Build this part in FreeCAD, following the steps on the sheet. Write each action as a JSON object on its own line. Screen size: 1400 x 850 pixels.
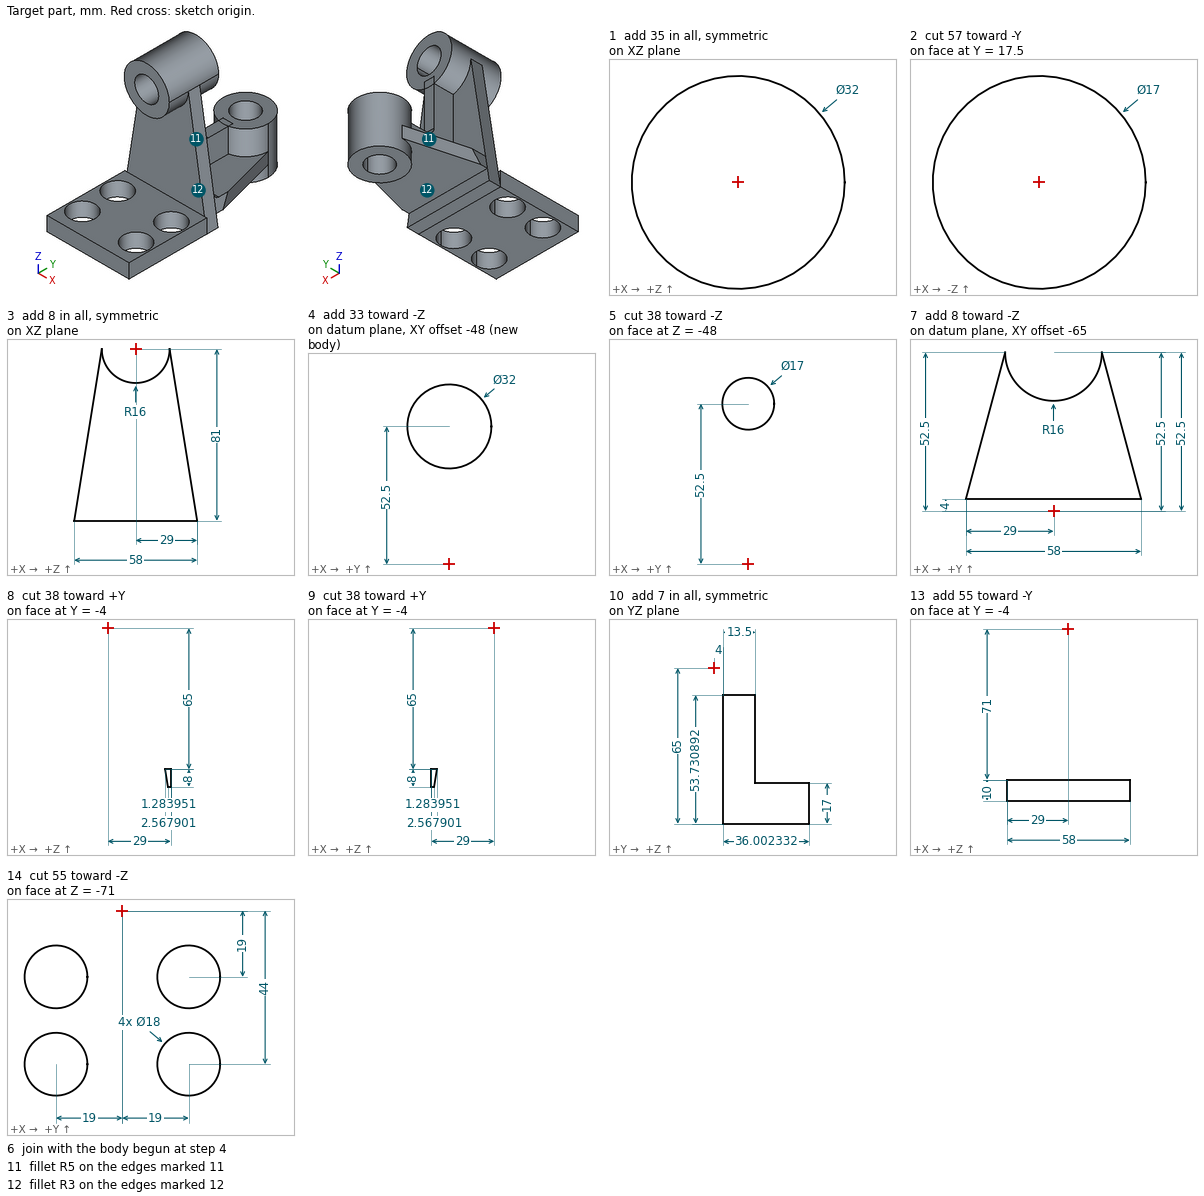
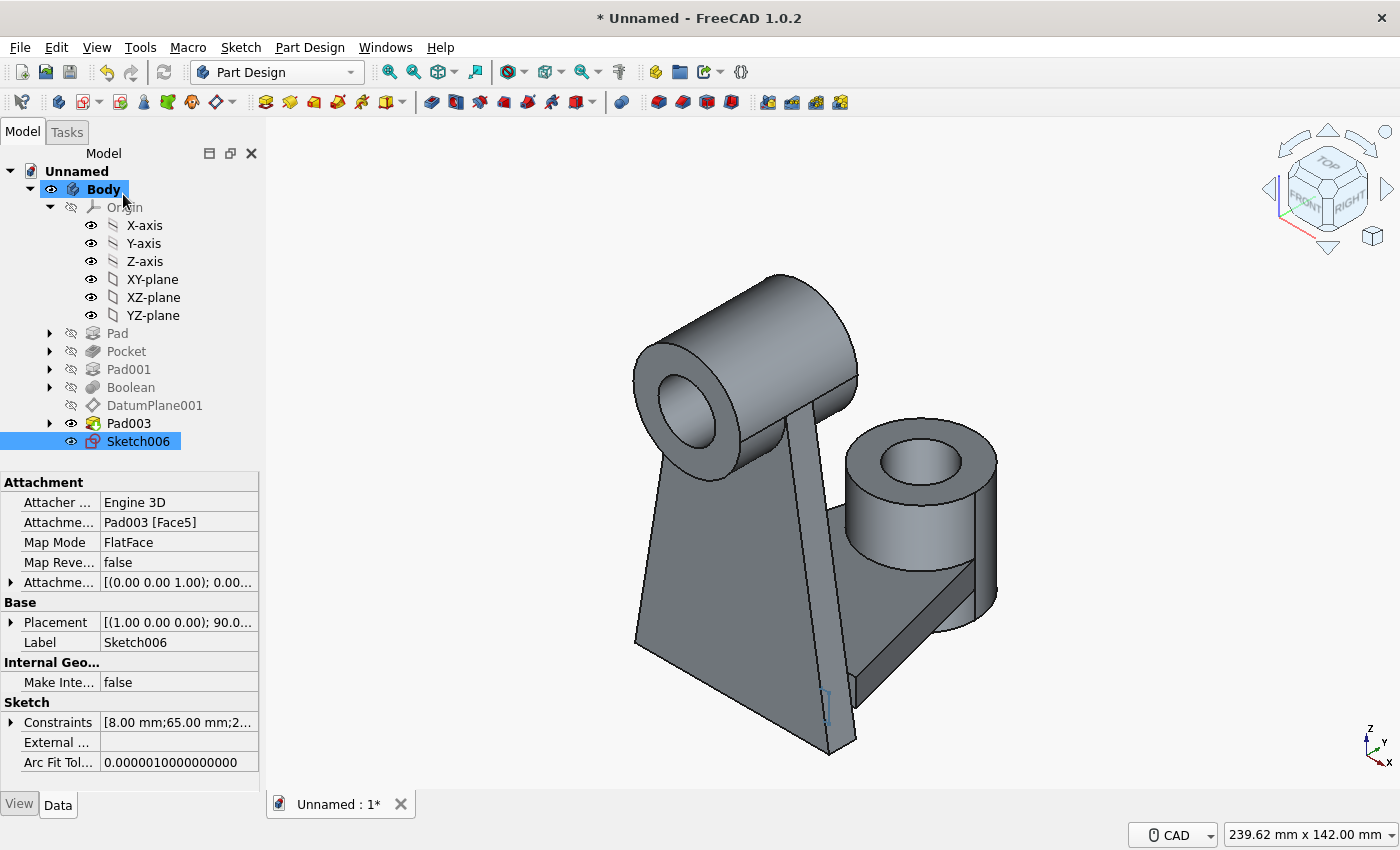
{"action": "left_click", "coordinate": [432, 102]}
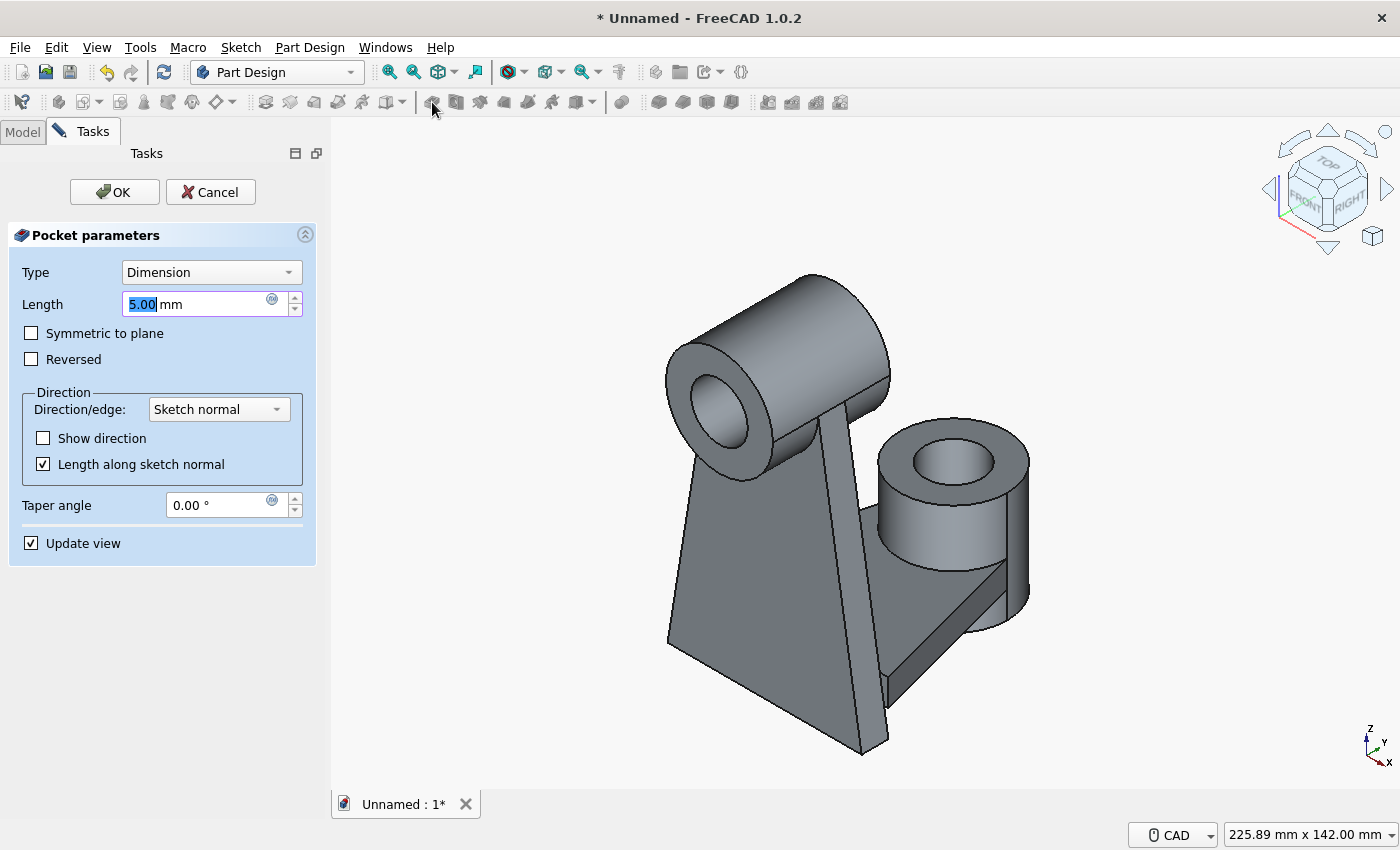
{"action": "type", "text": "38"}
{"action": "key", "text": "Tab"}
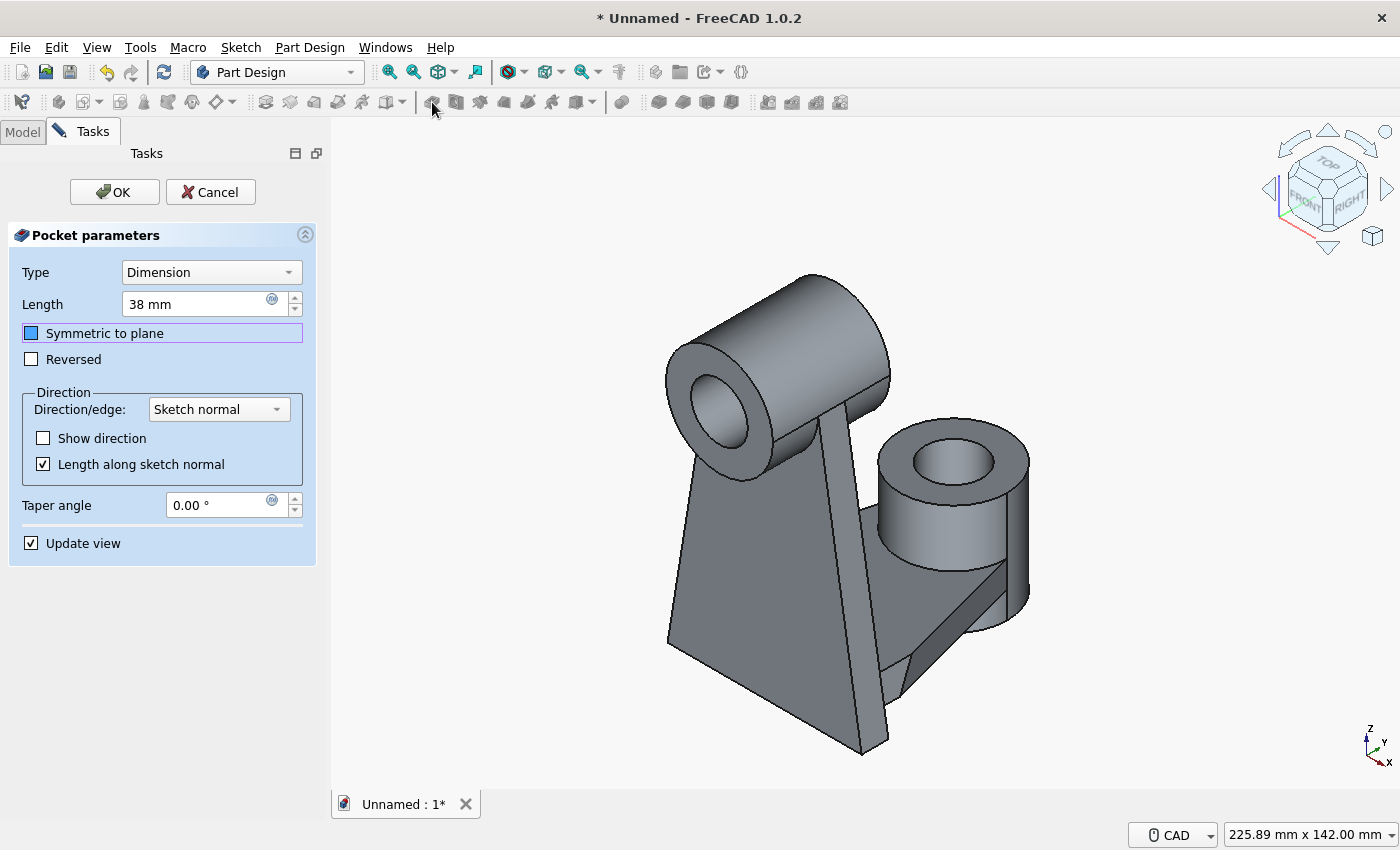
{"action": "left_click", "coordinate": [115, 192]}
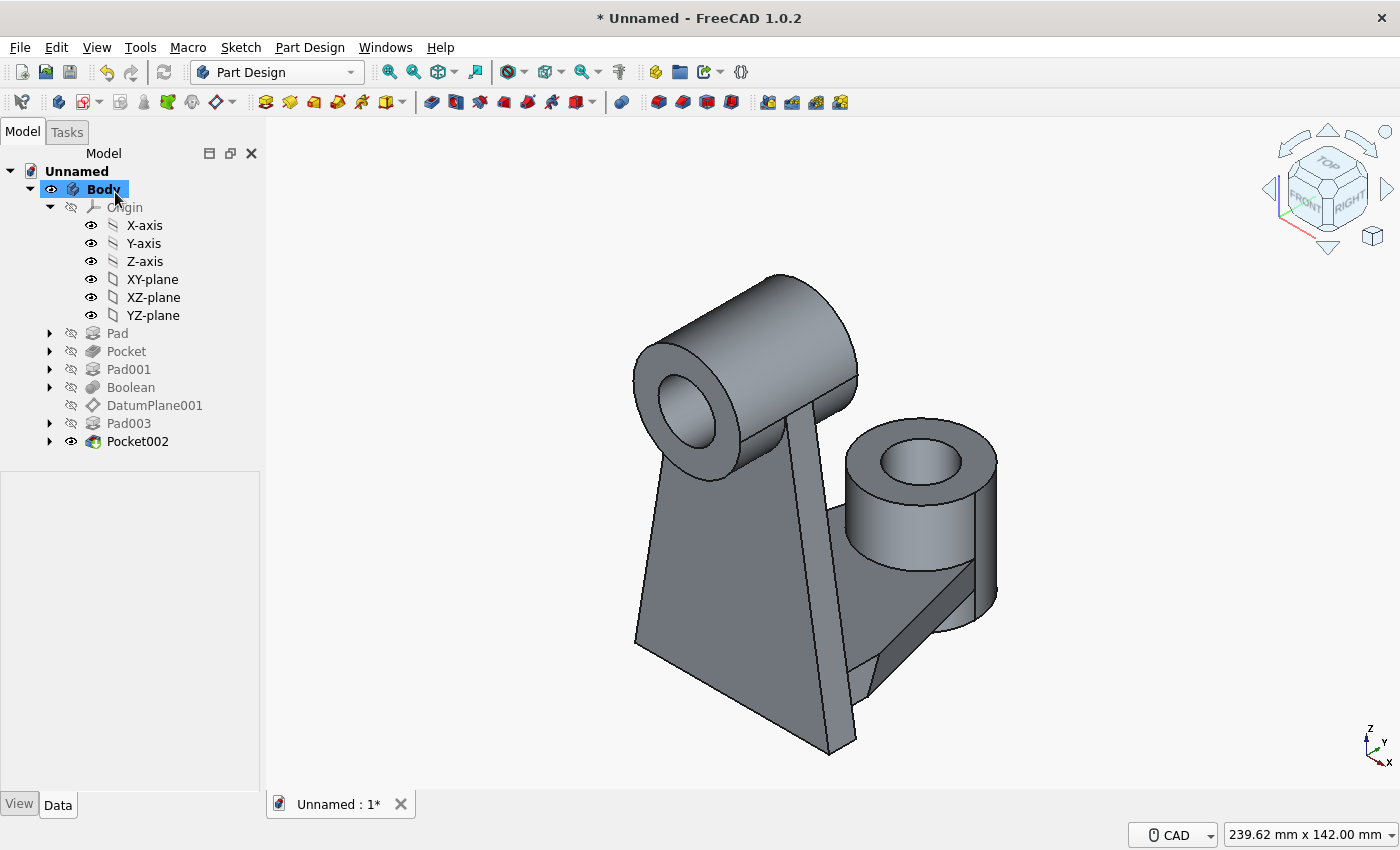
{"action": "left_click", "coordinate": [732, 586]}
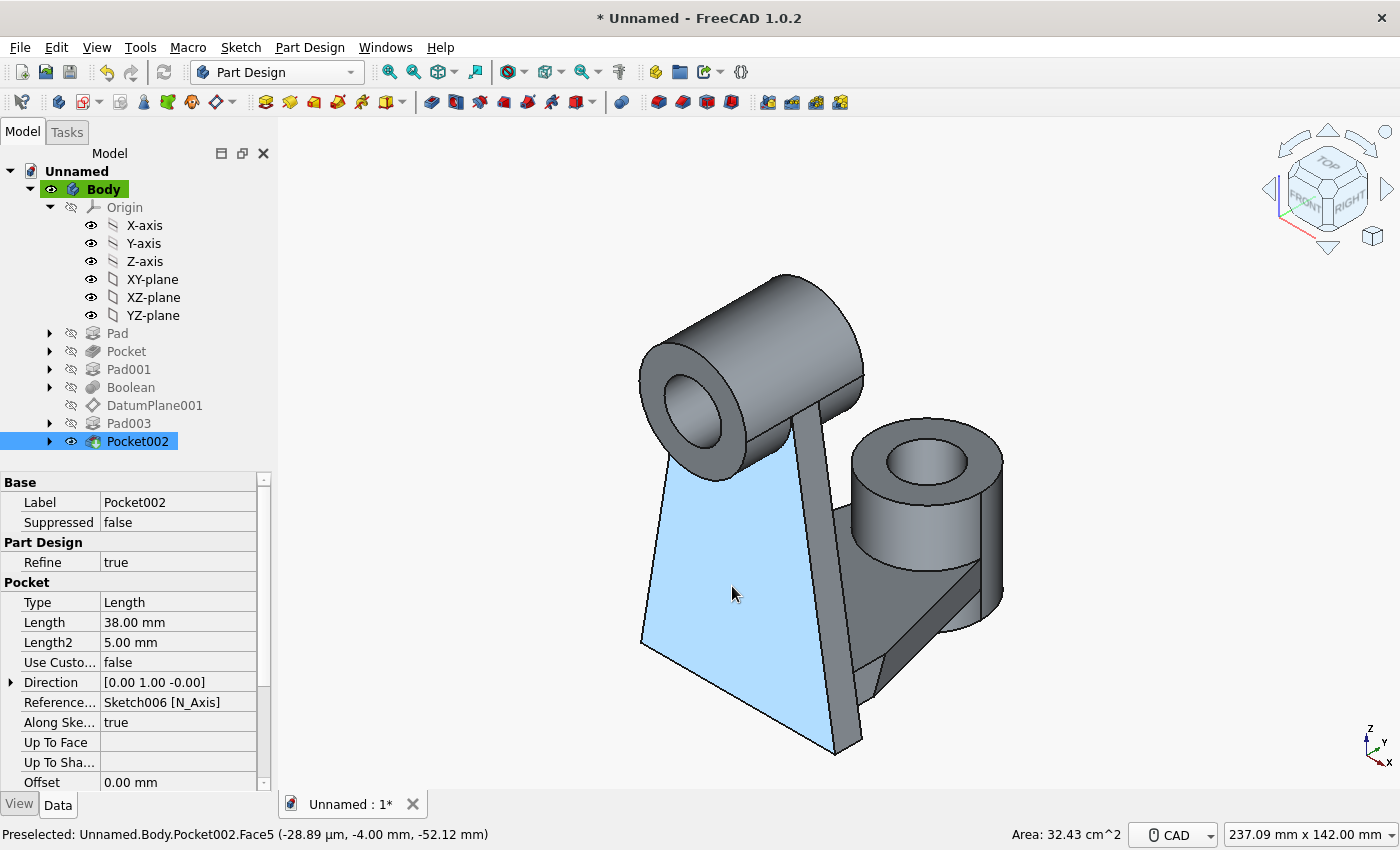
{"action": "left_click", "coordinate": [84, 102]}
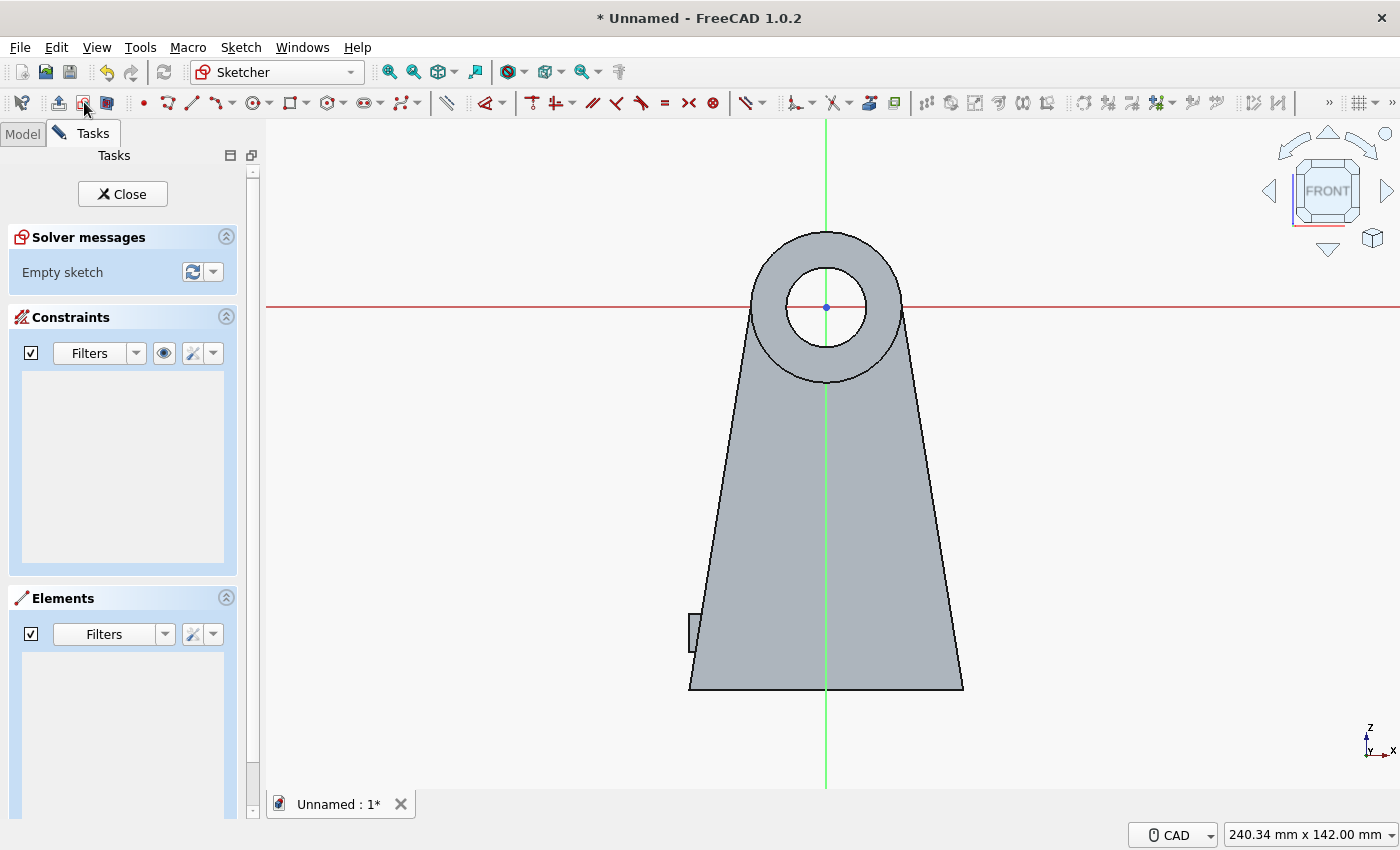
{"action": "left_click", "coordinate": [108, 104]}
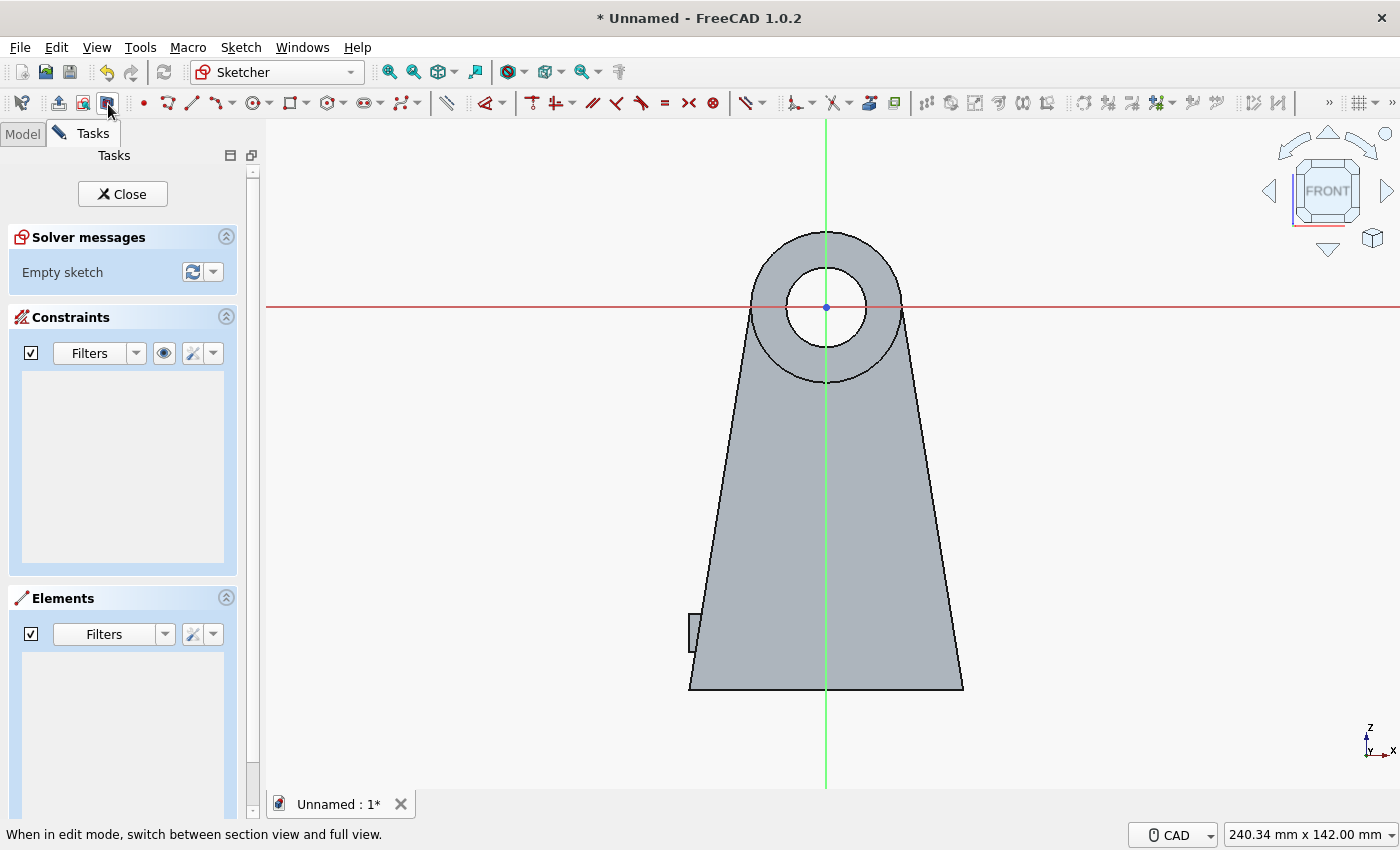
{"action": "scroll", "coordinate": [689, 651], "scroll_direction": "up", "scroll_amount": 12}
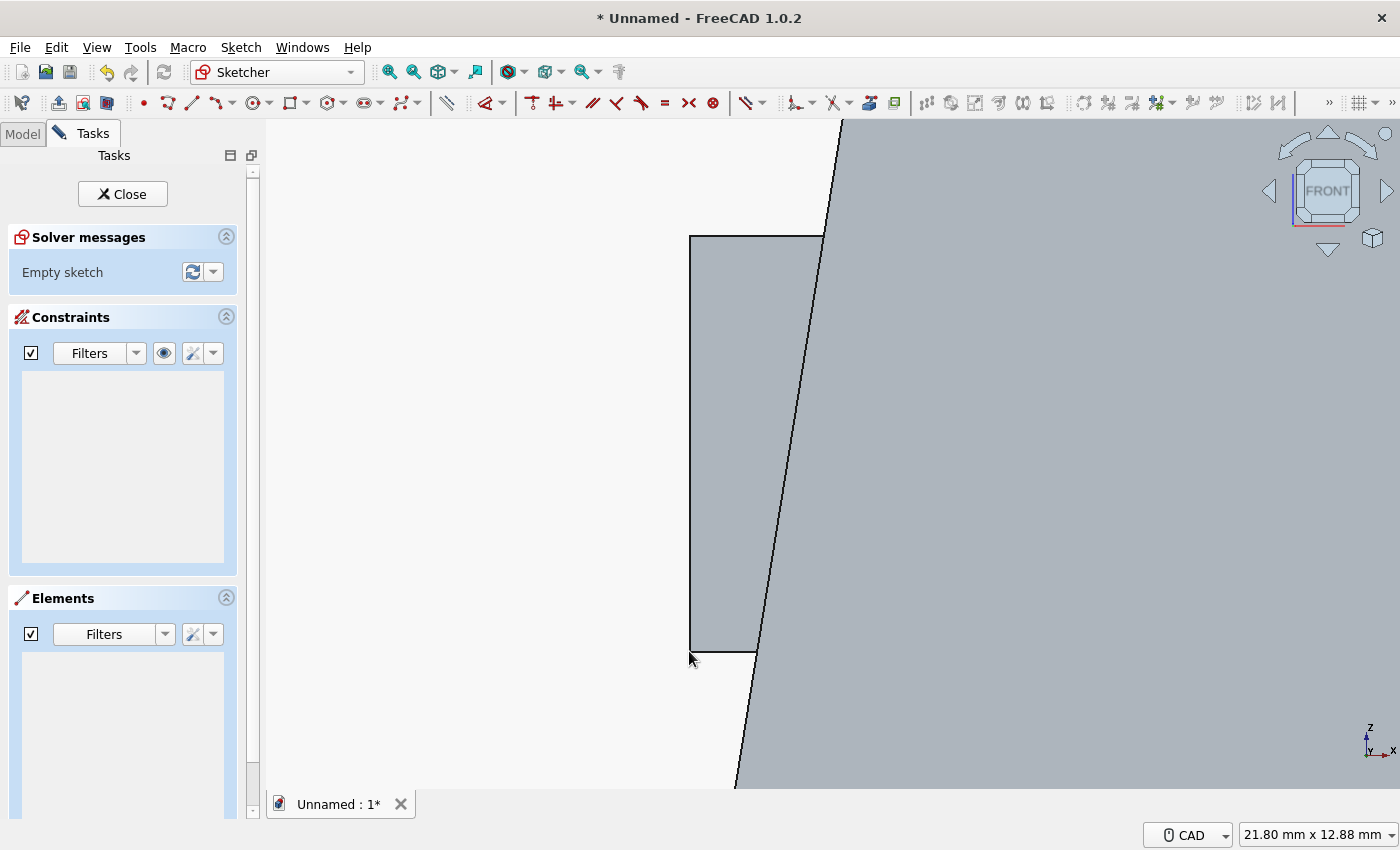
{"action": "key", "text": "g m"}